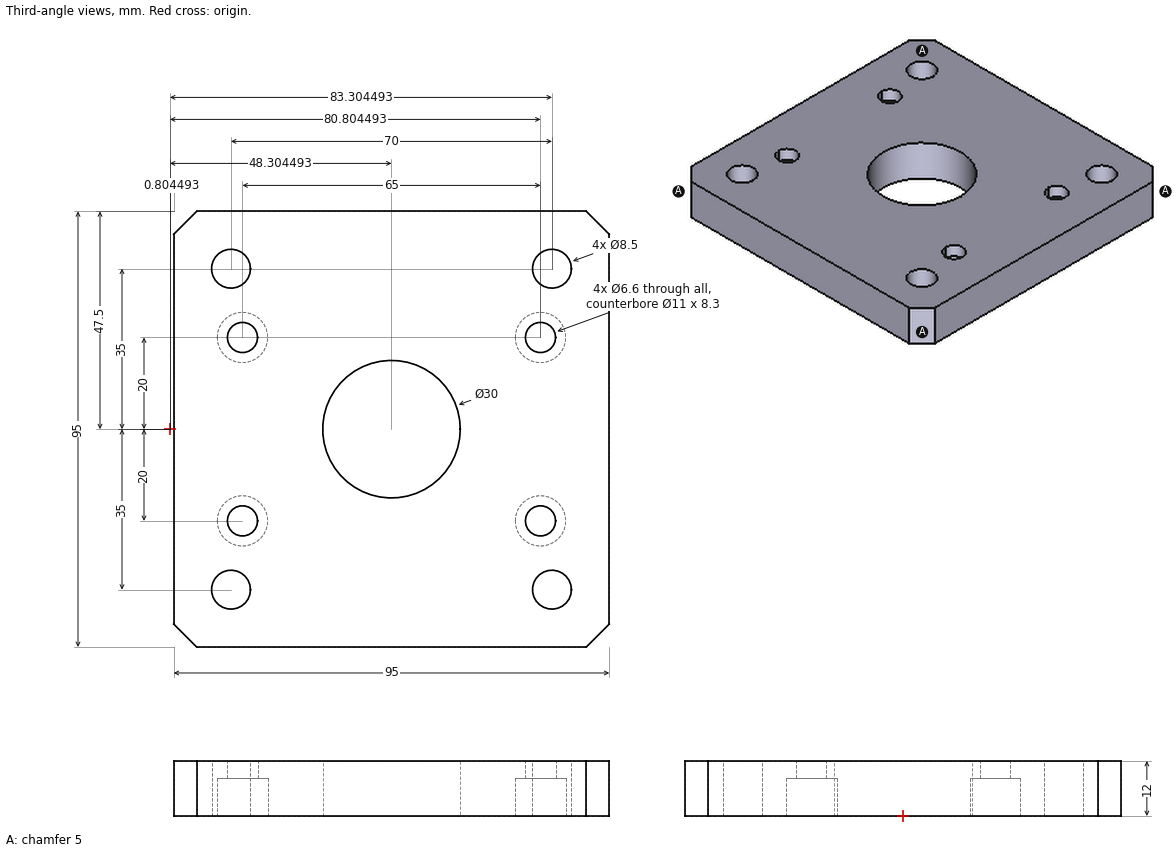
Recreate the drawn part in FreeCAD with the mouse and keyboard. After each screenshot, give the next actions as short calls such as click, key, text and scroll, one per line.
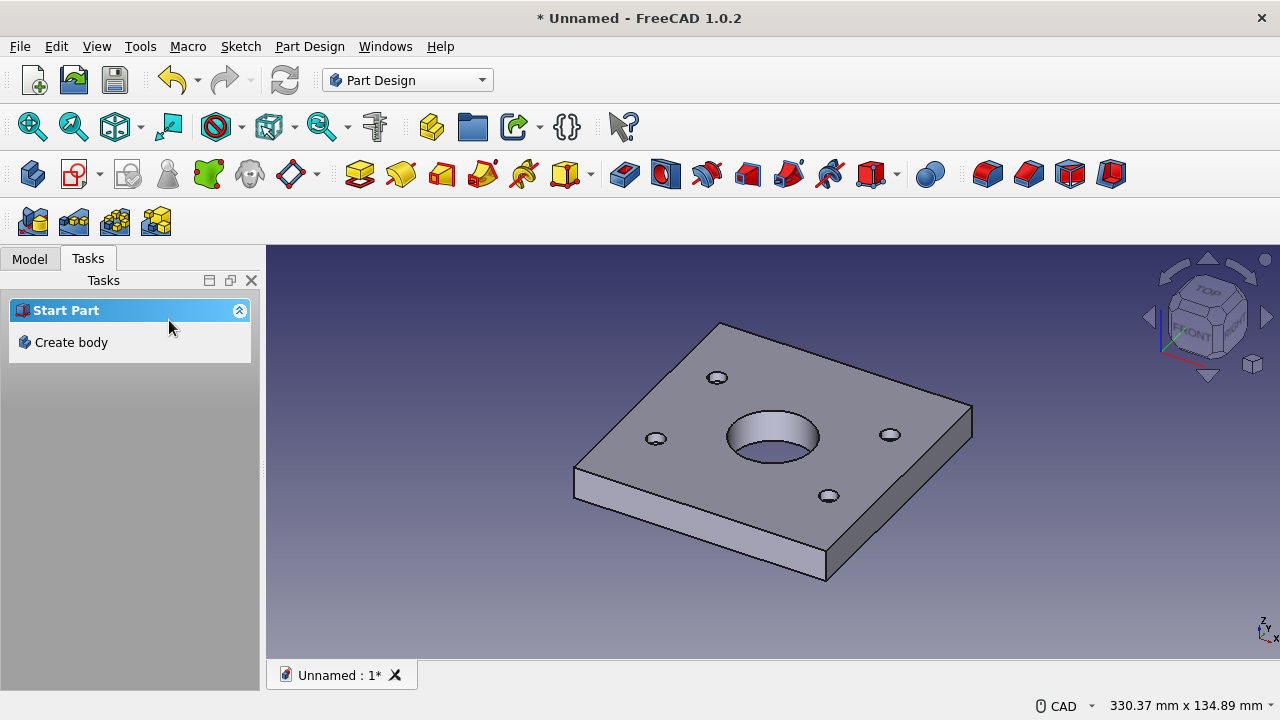
click(74, 174)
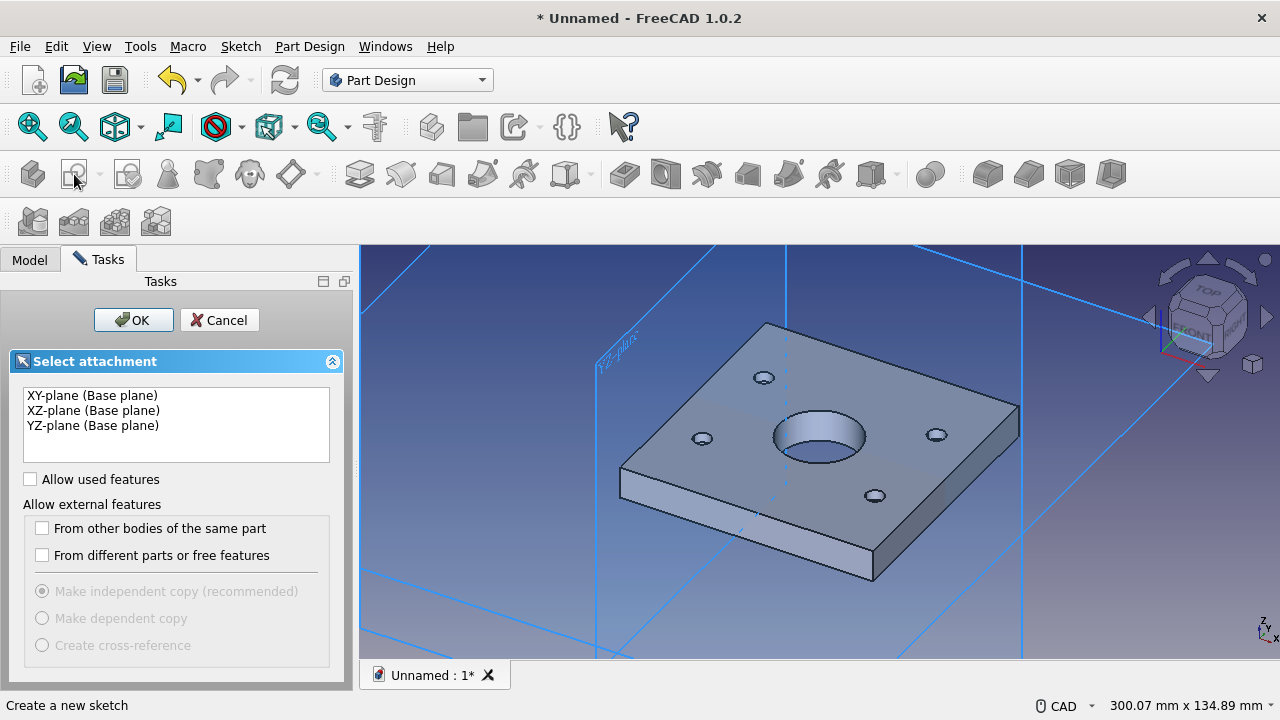
click(84, 396)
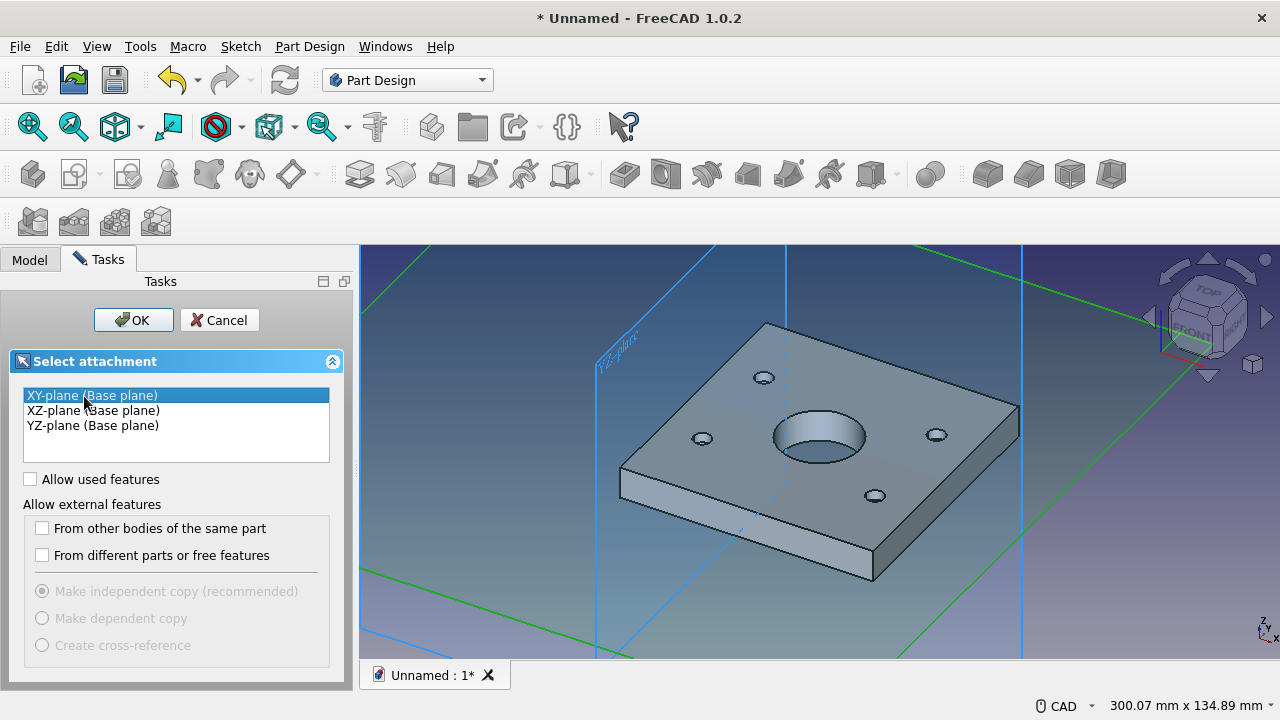
click(134, 320)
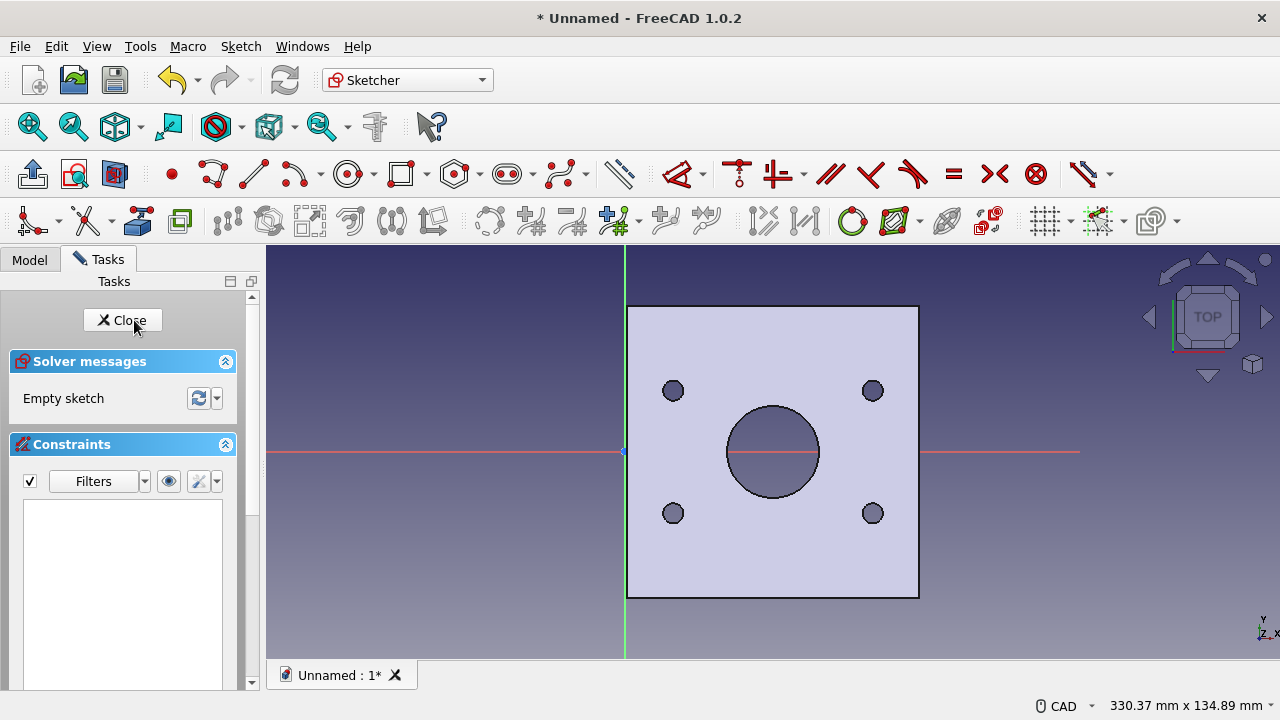
click(115, 174)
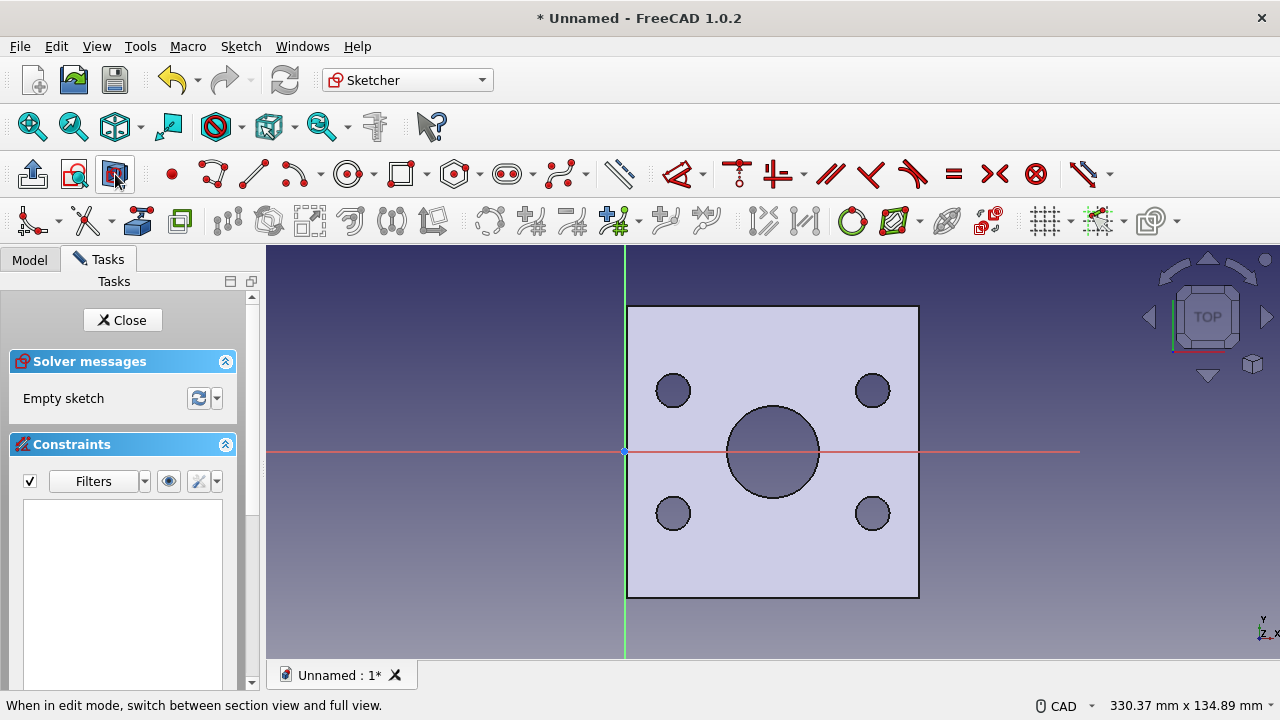
click(348, 174)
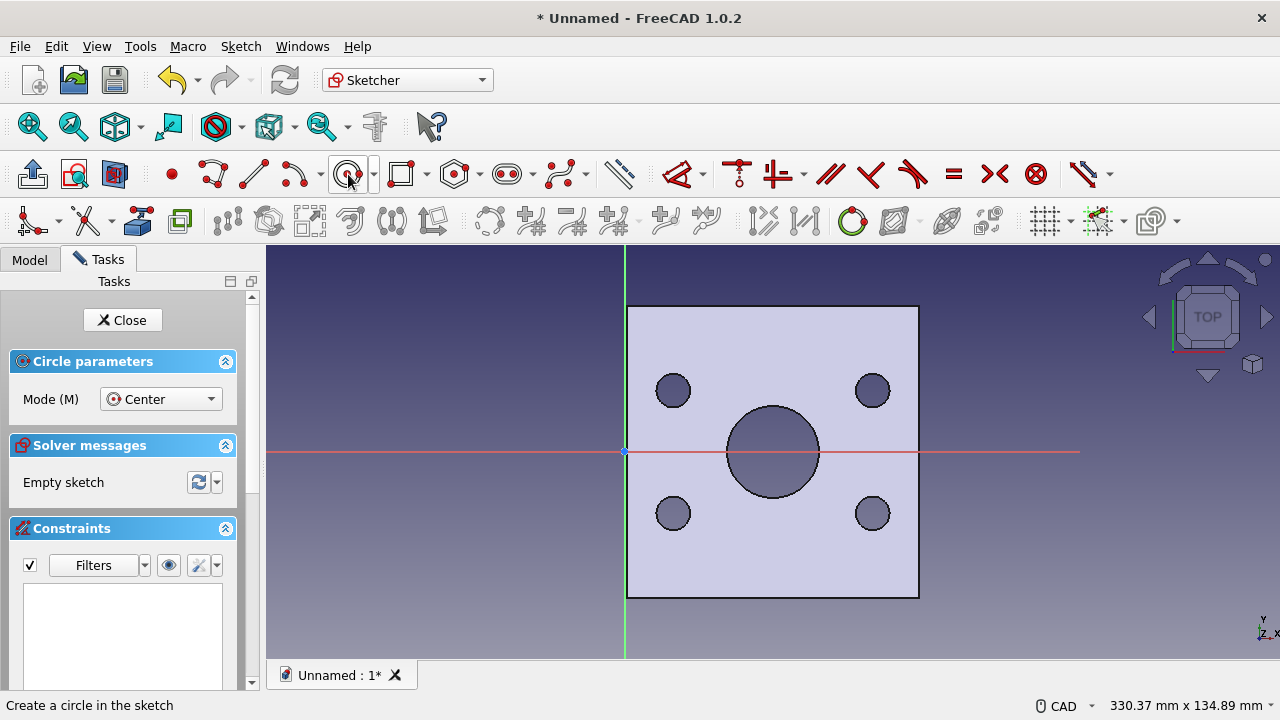
scroll(880, 345, up, 3)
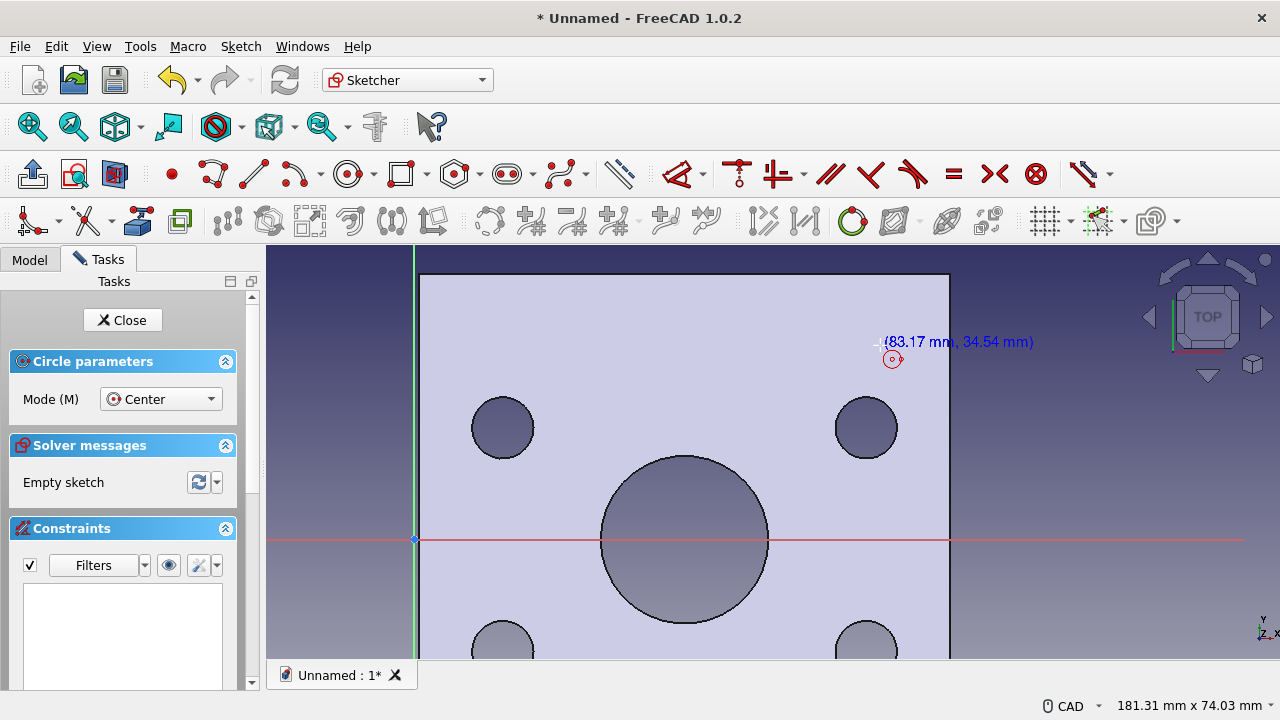
click(880, 344)
click(897, 327)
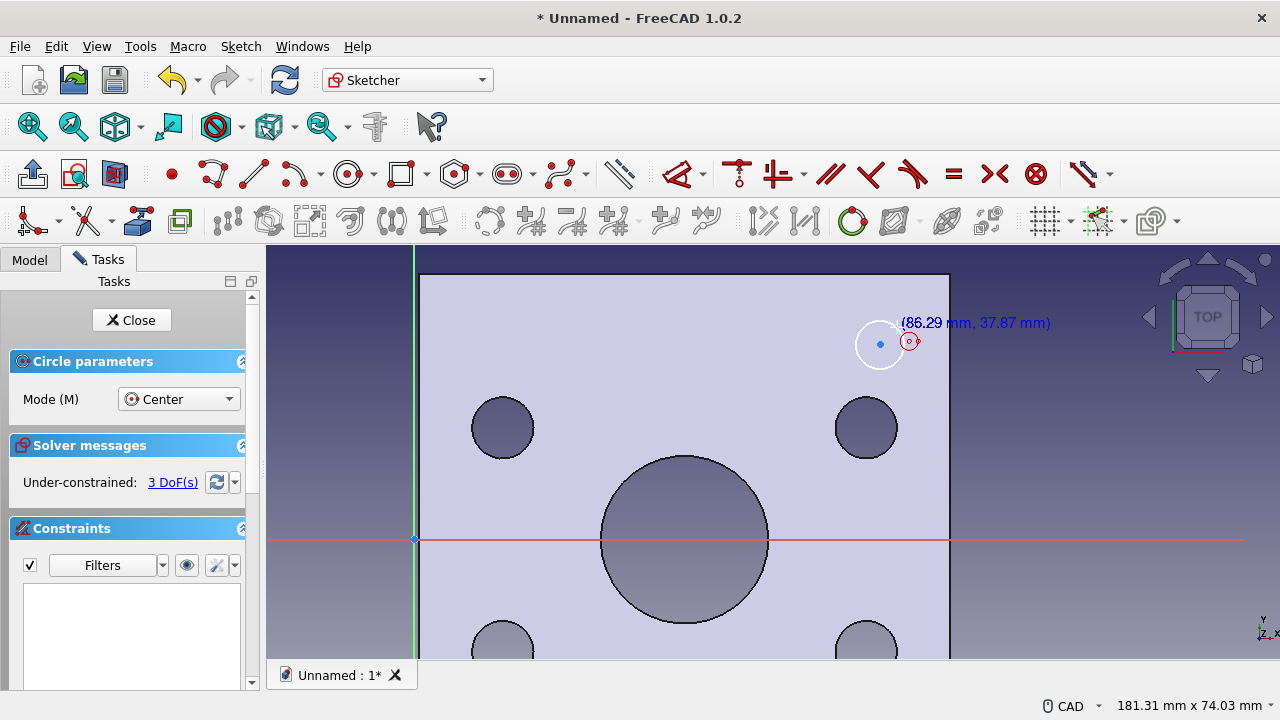
click(489, 344)
click(506, 327)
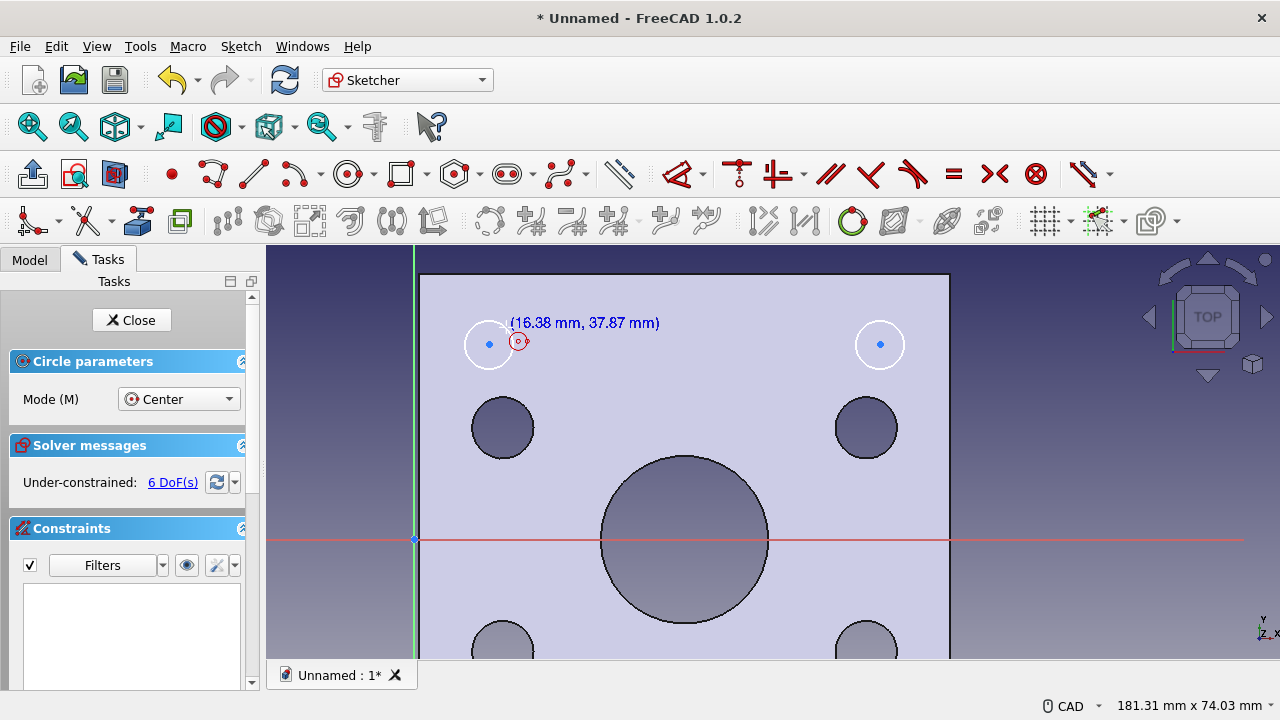
scroll(760, 345, down, 3)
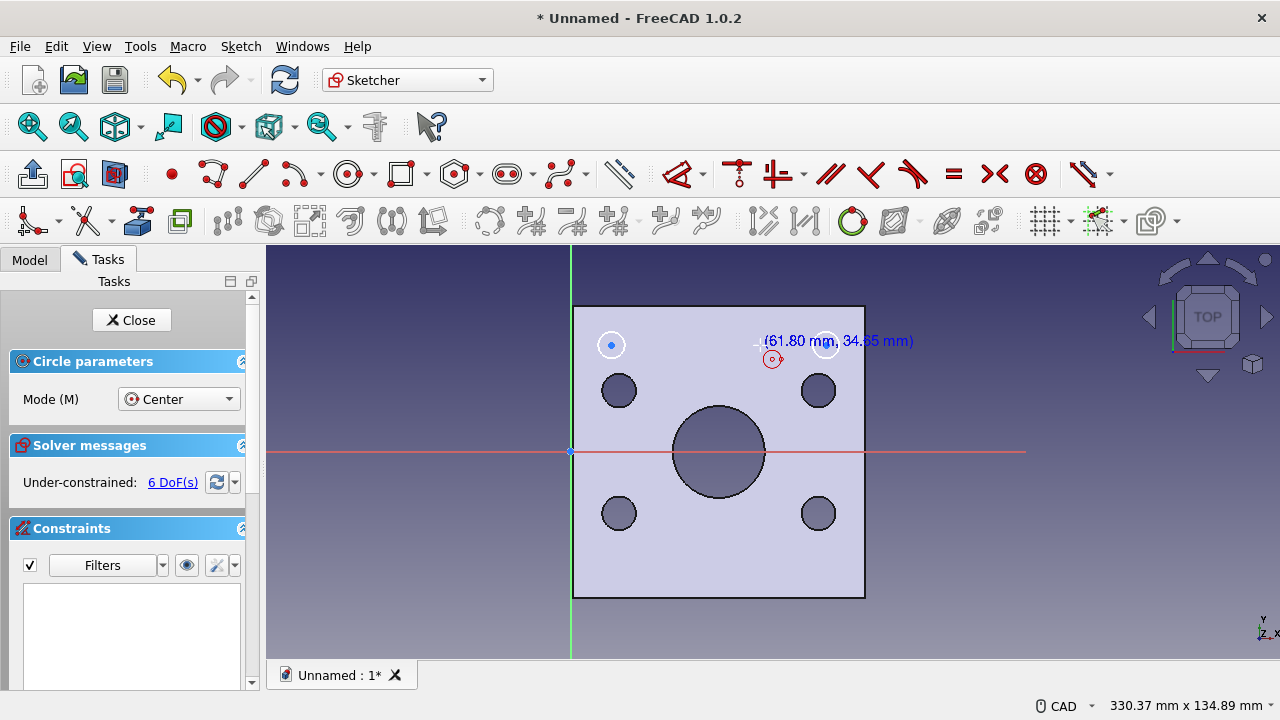
scroll(611, 559, up, 3)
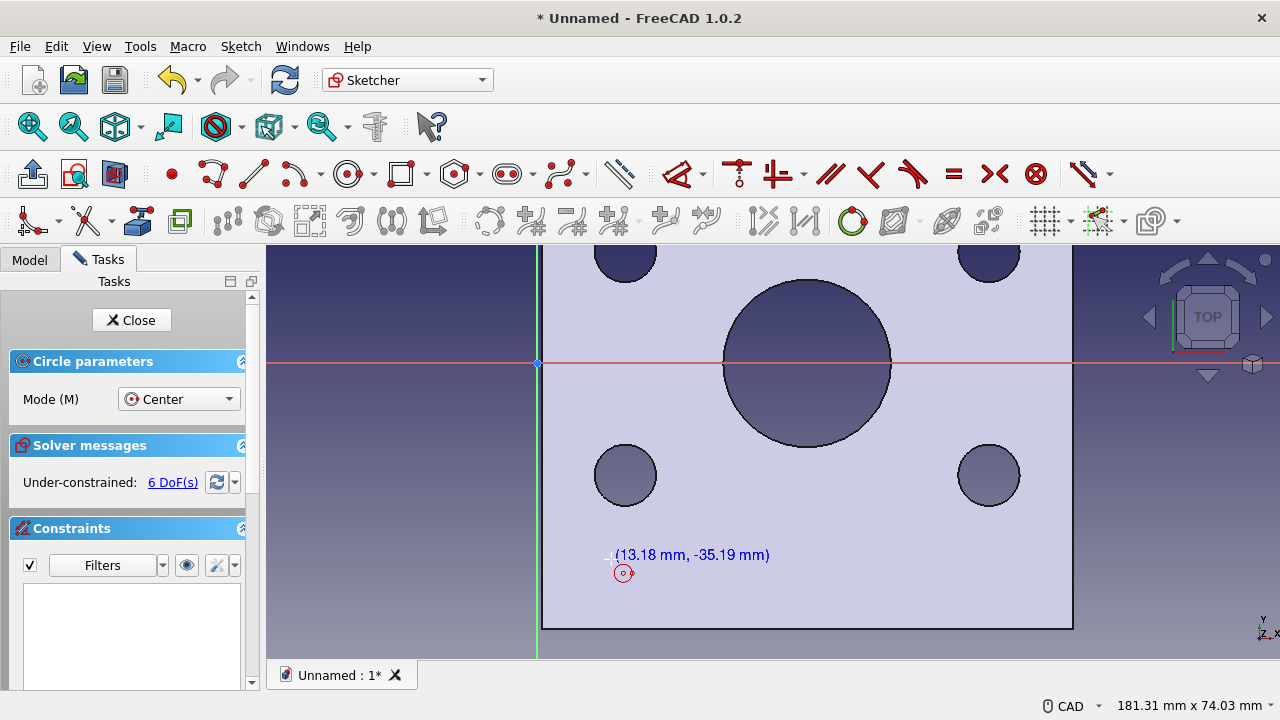
click(611, 559)
click(628, 542)